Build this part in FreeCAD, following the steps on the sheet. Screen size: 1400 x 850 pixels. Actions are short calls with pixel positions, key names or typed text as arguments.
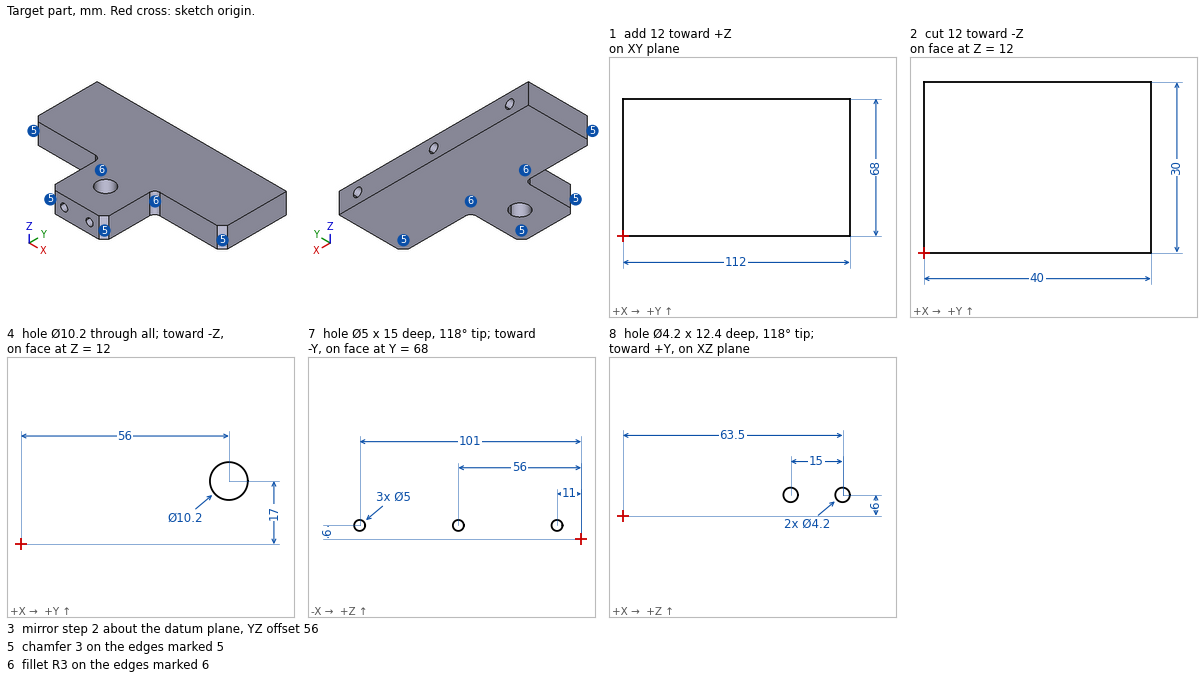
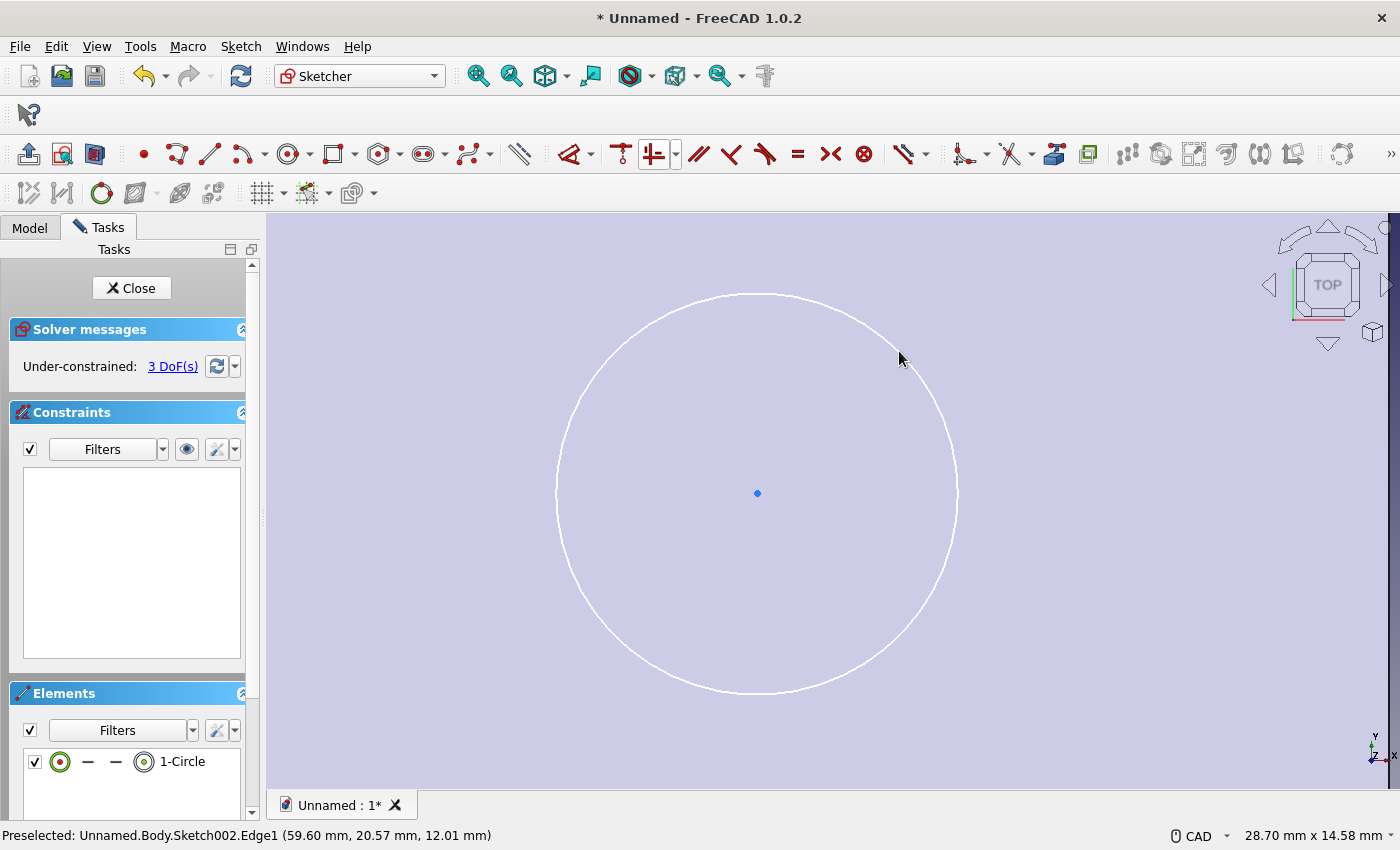
key(d)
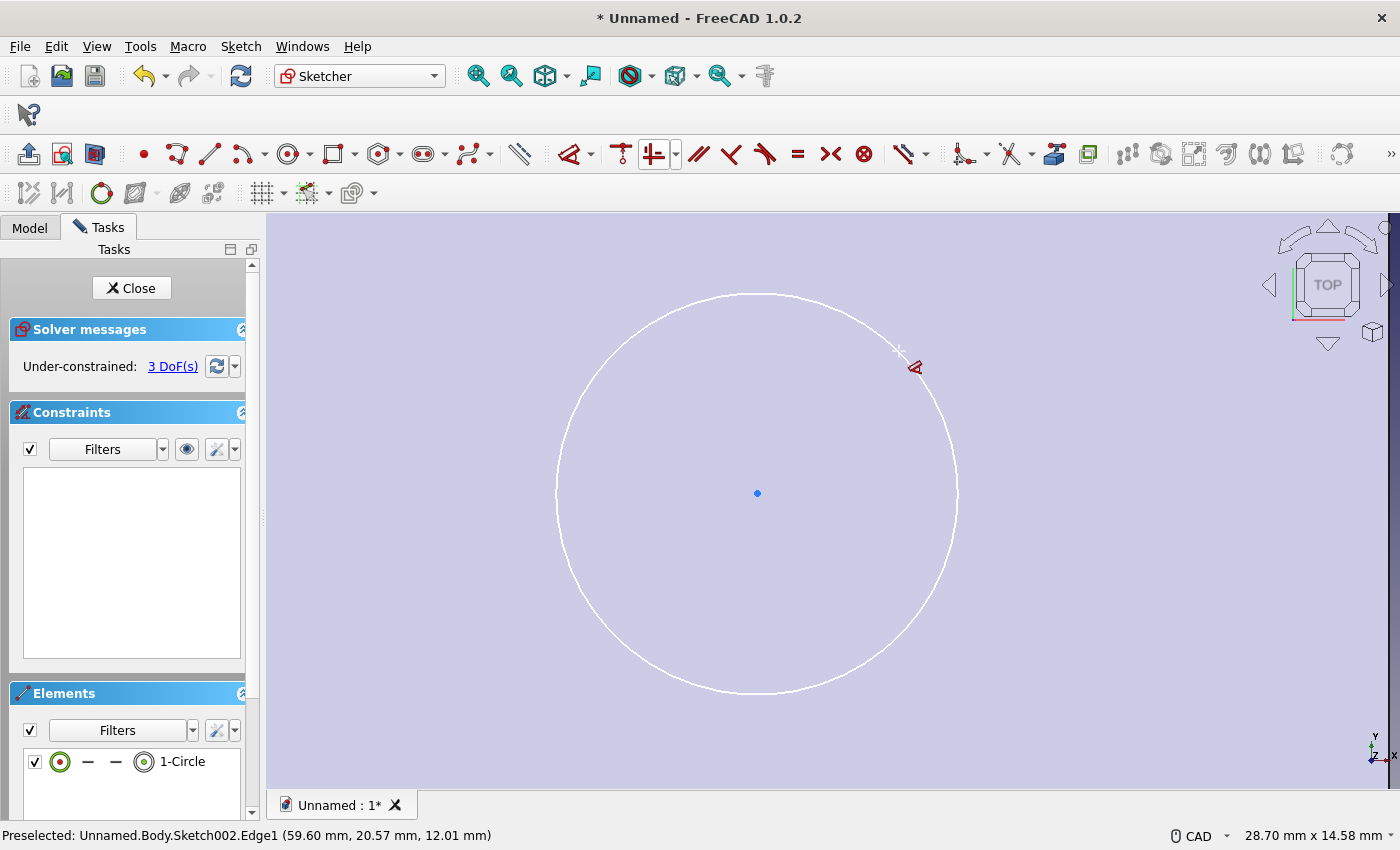
click(899, 352)
click(922, 329)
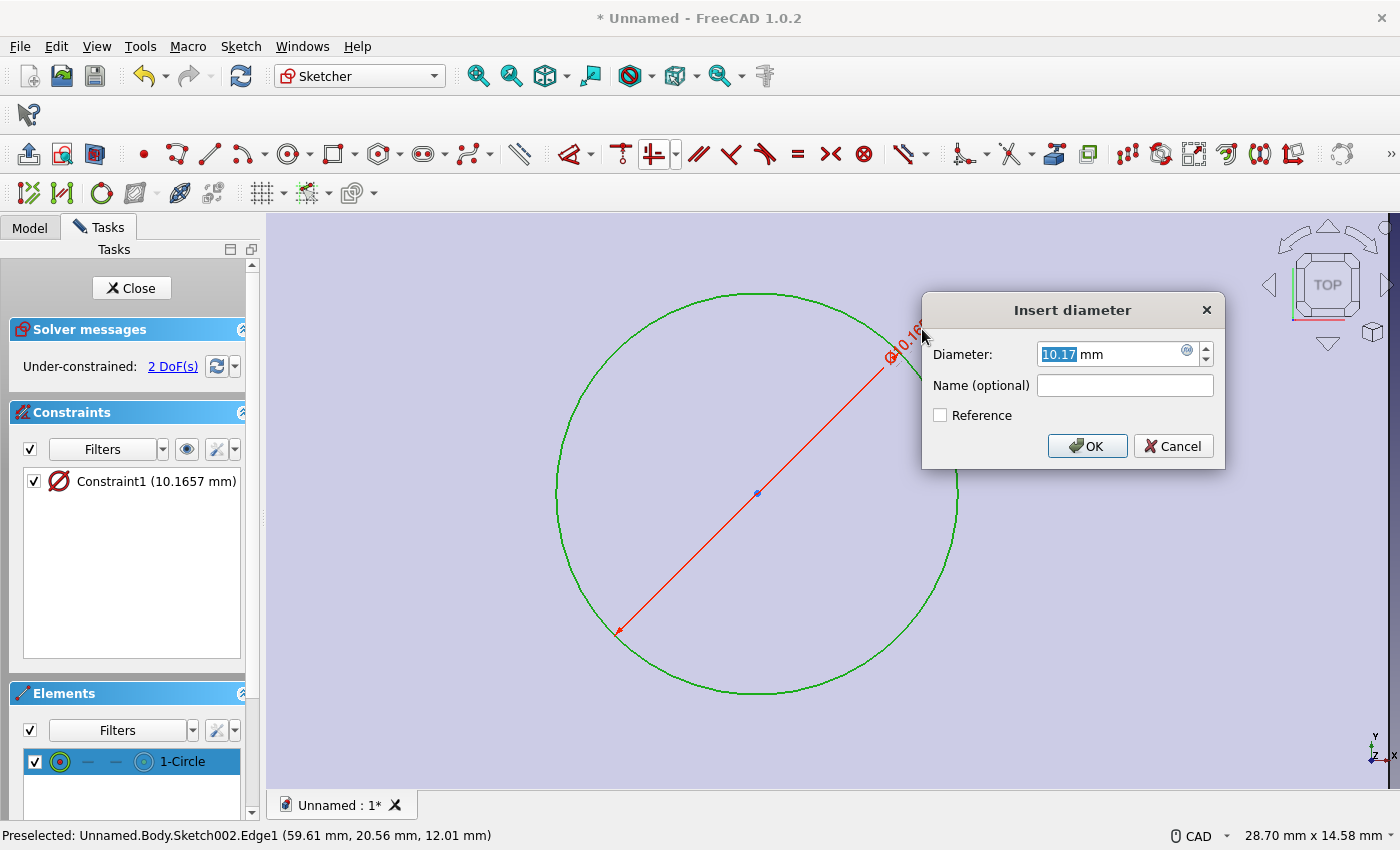
text(10.2)
key(Return)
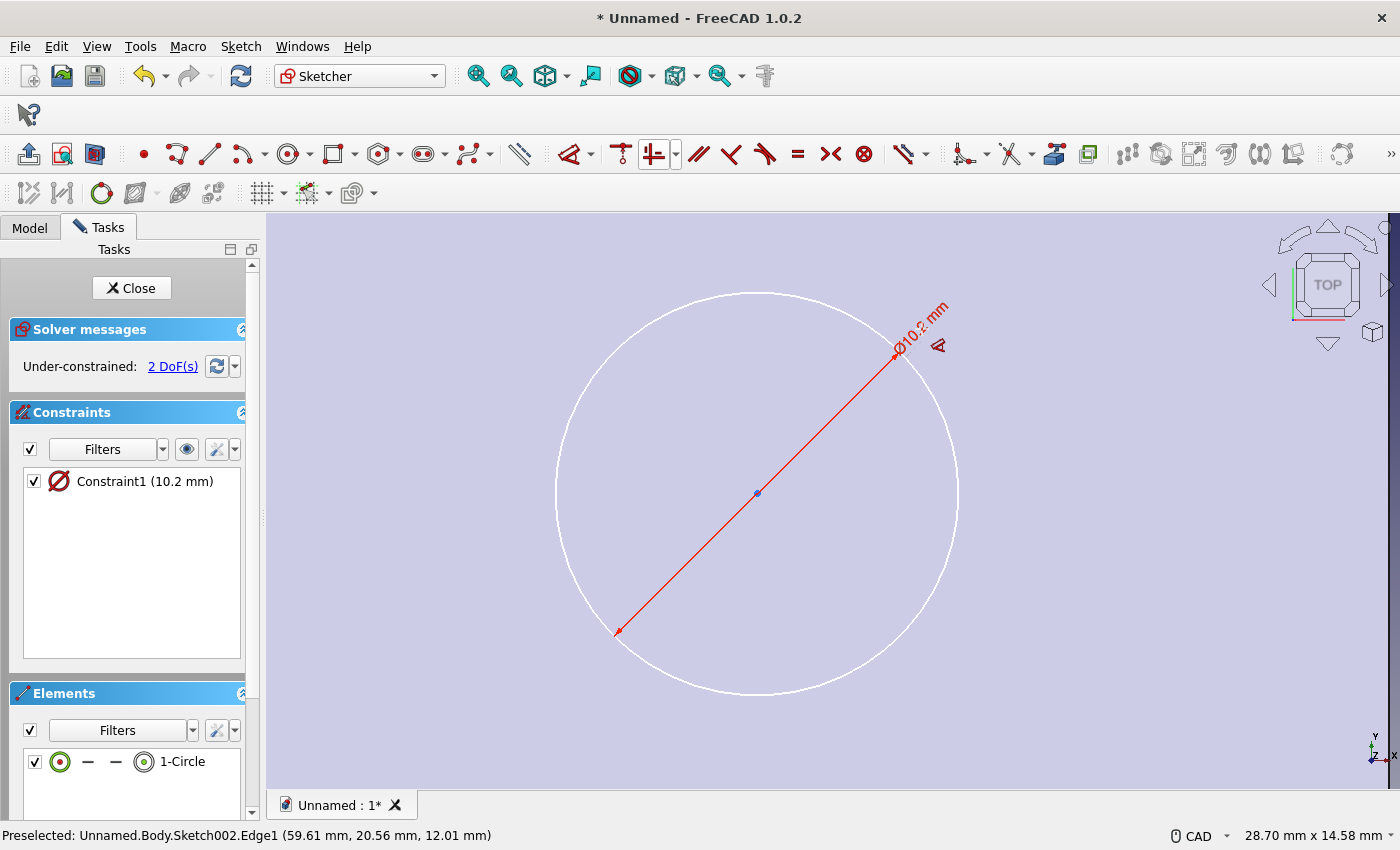
click(757, 494)
click(525, 460)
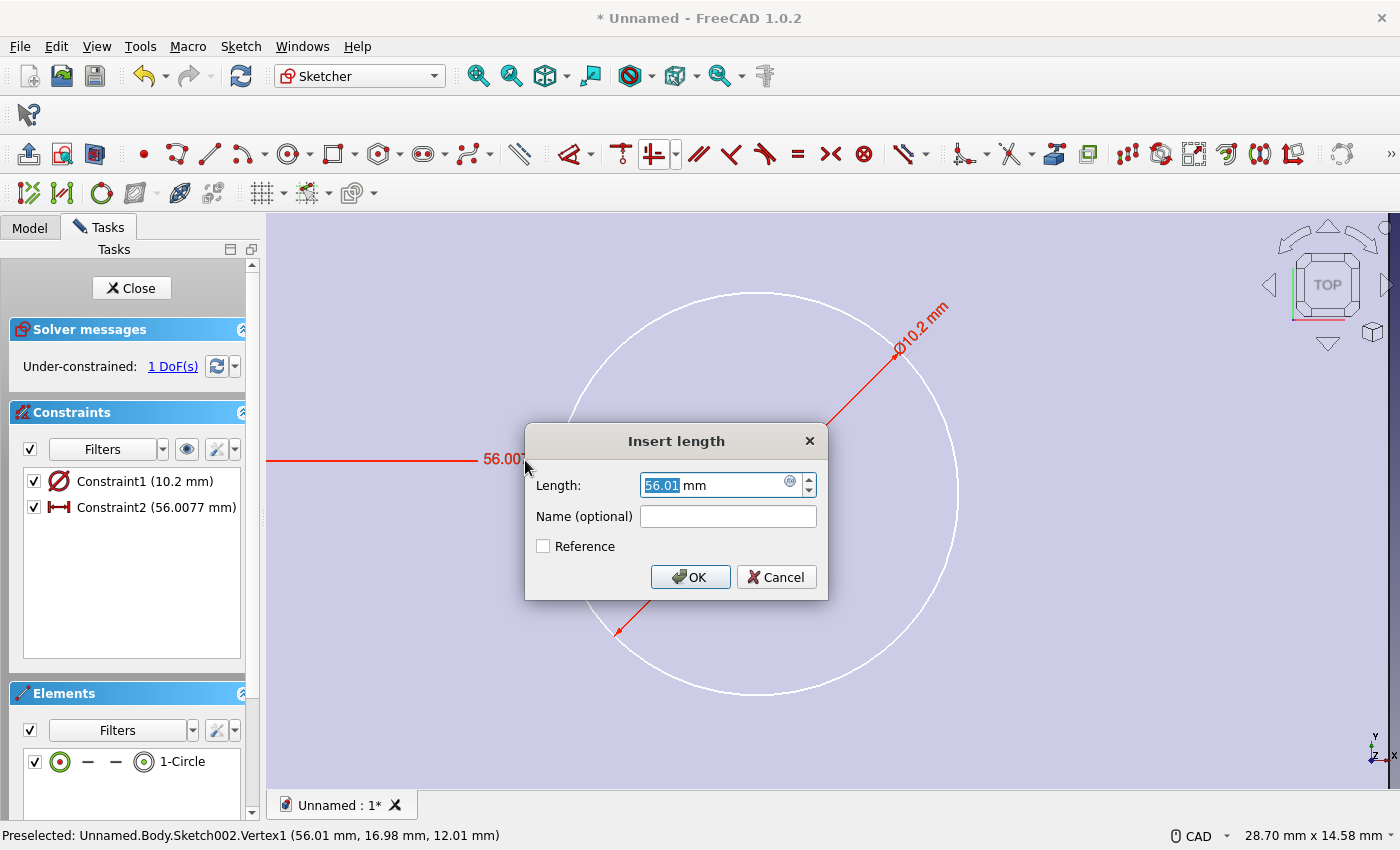
text(56)
key(Return)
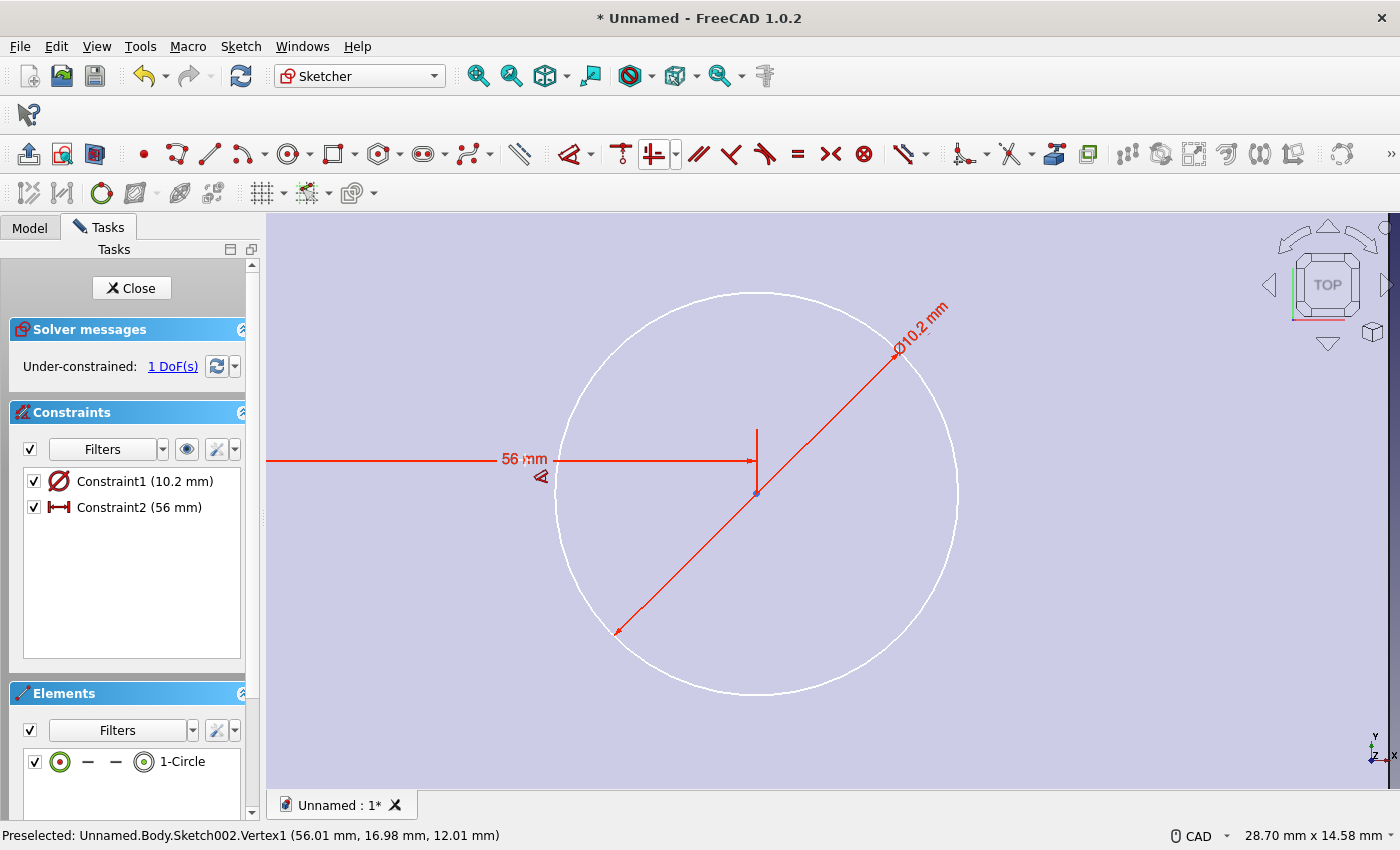
click(757, 494)
click(791, 627)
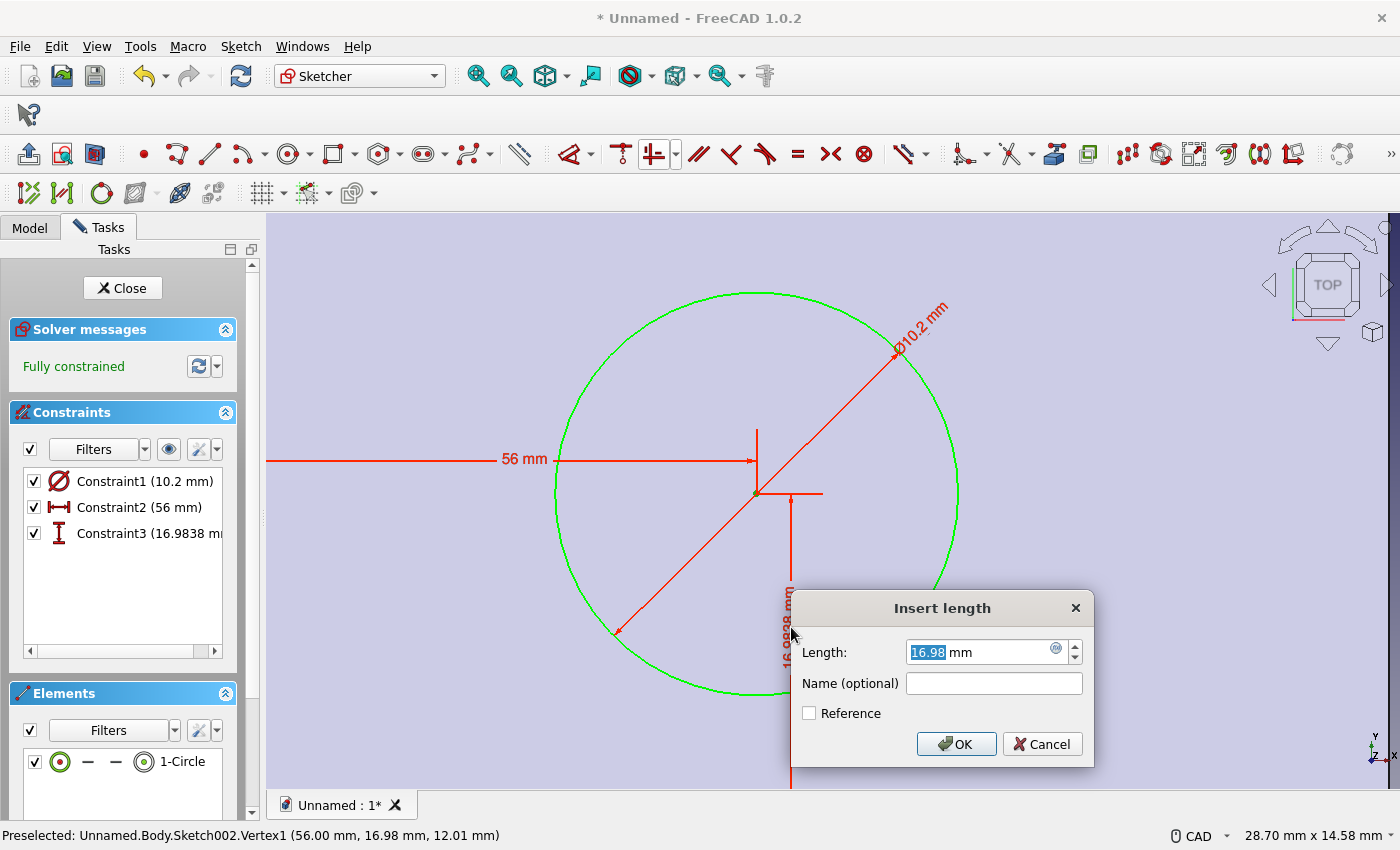
text(17)
key(Return)
key(Escape)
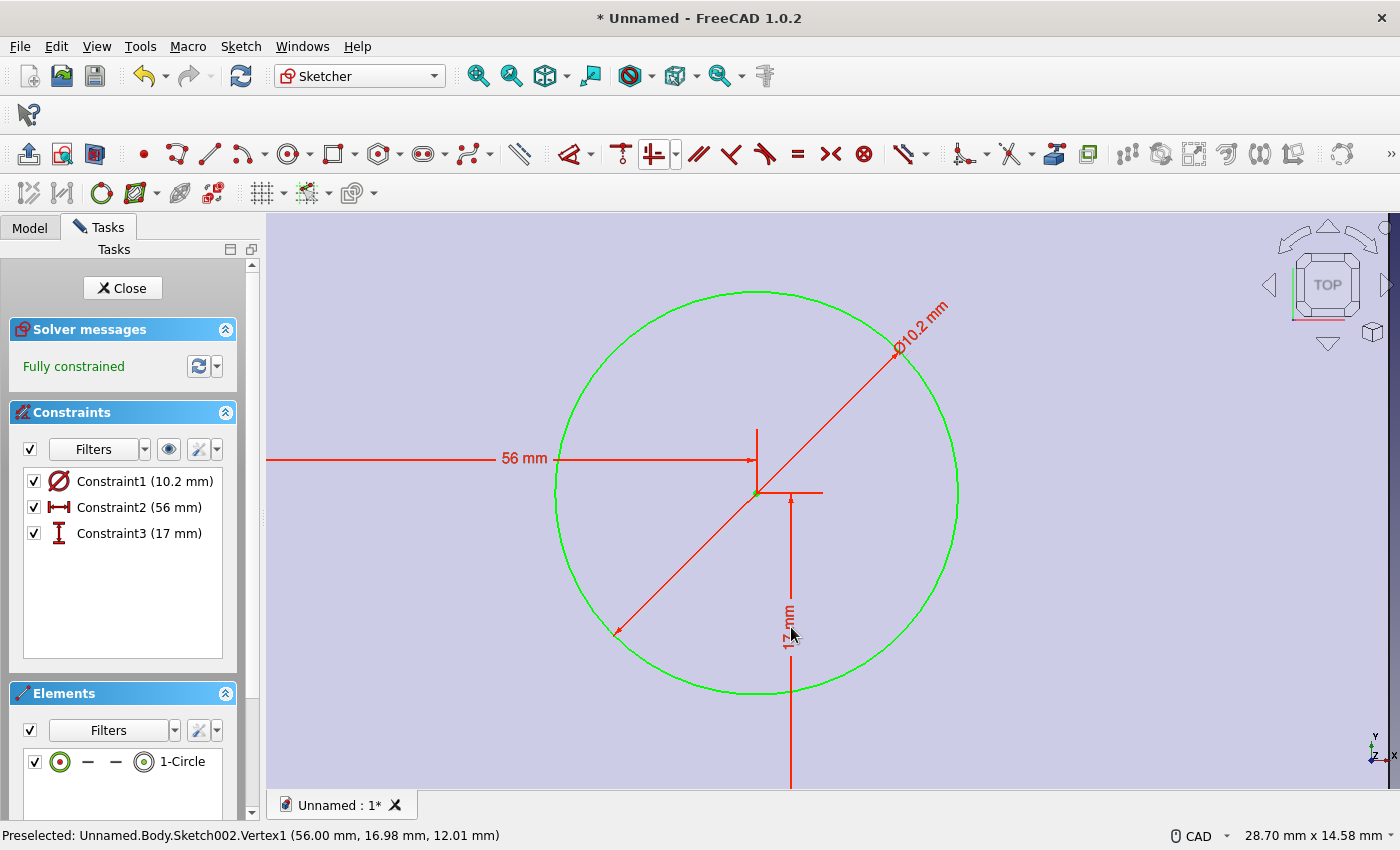
click(123, 288)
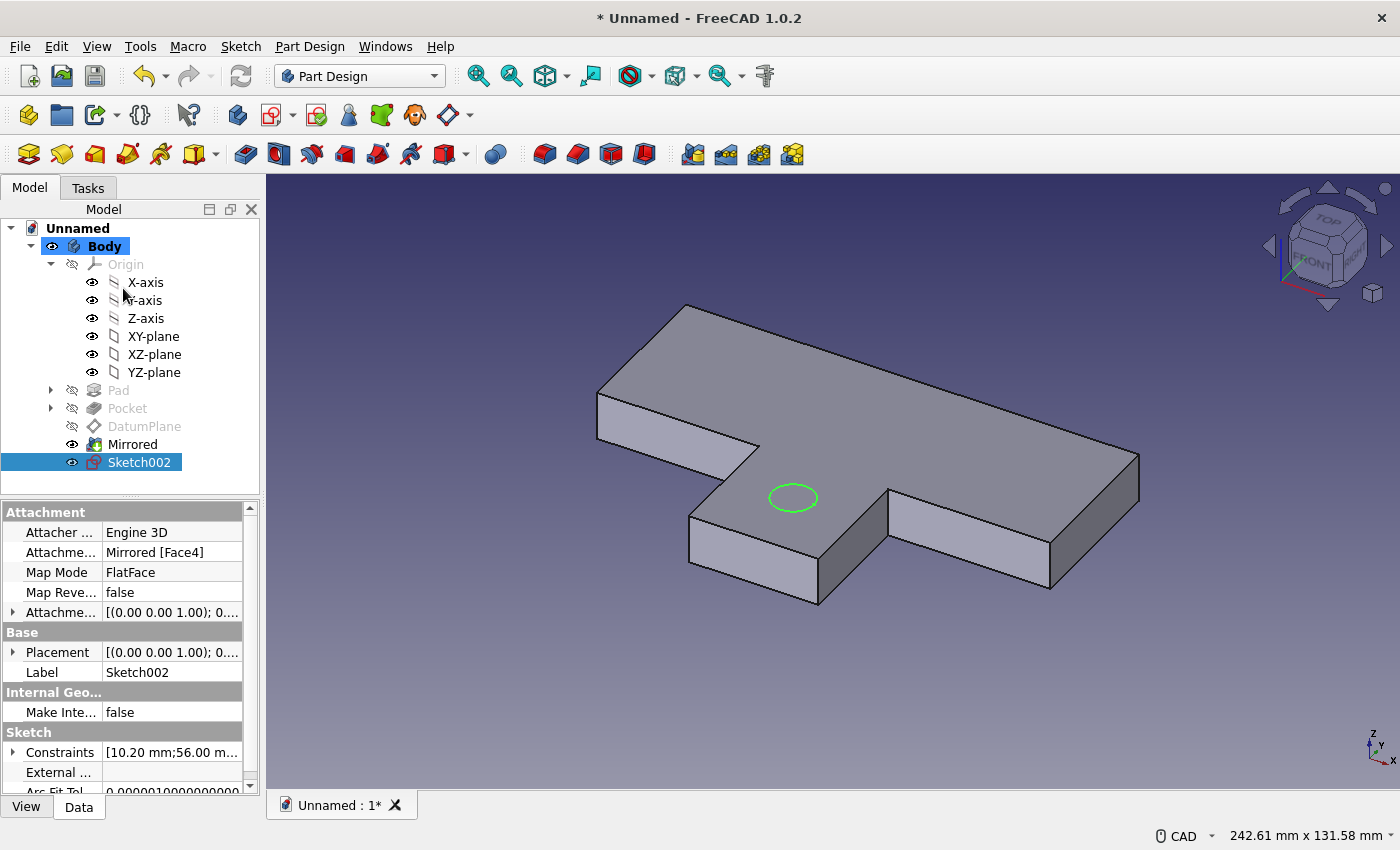
click(279, 154)